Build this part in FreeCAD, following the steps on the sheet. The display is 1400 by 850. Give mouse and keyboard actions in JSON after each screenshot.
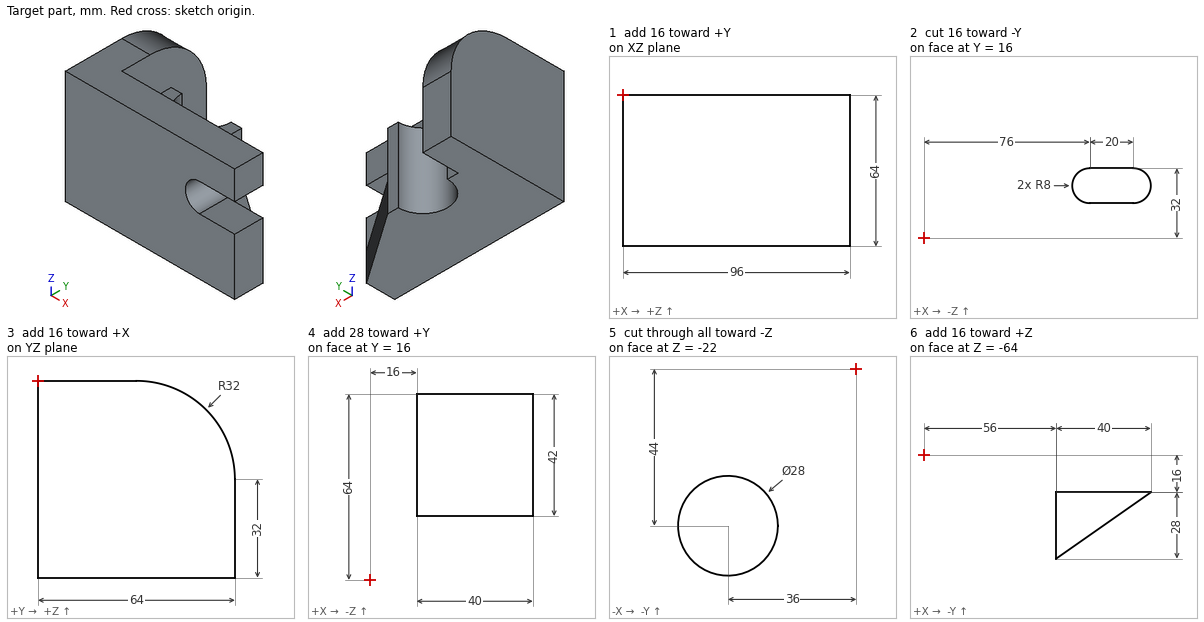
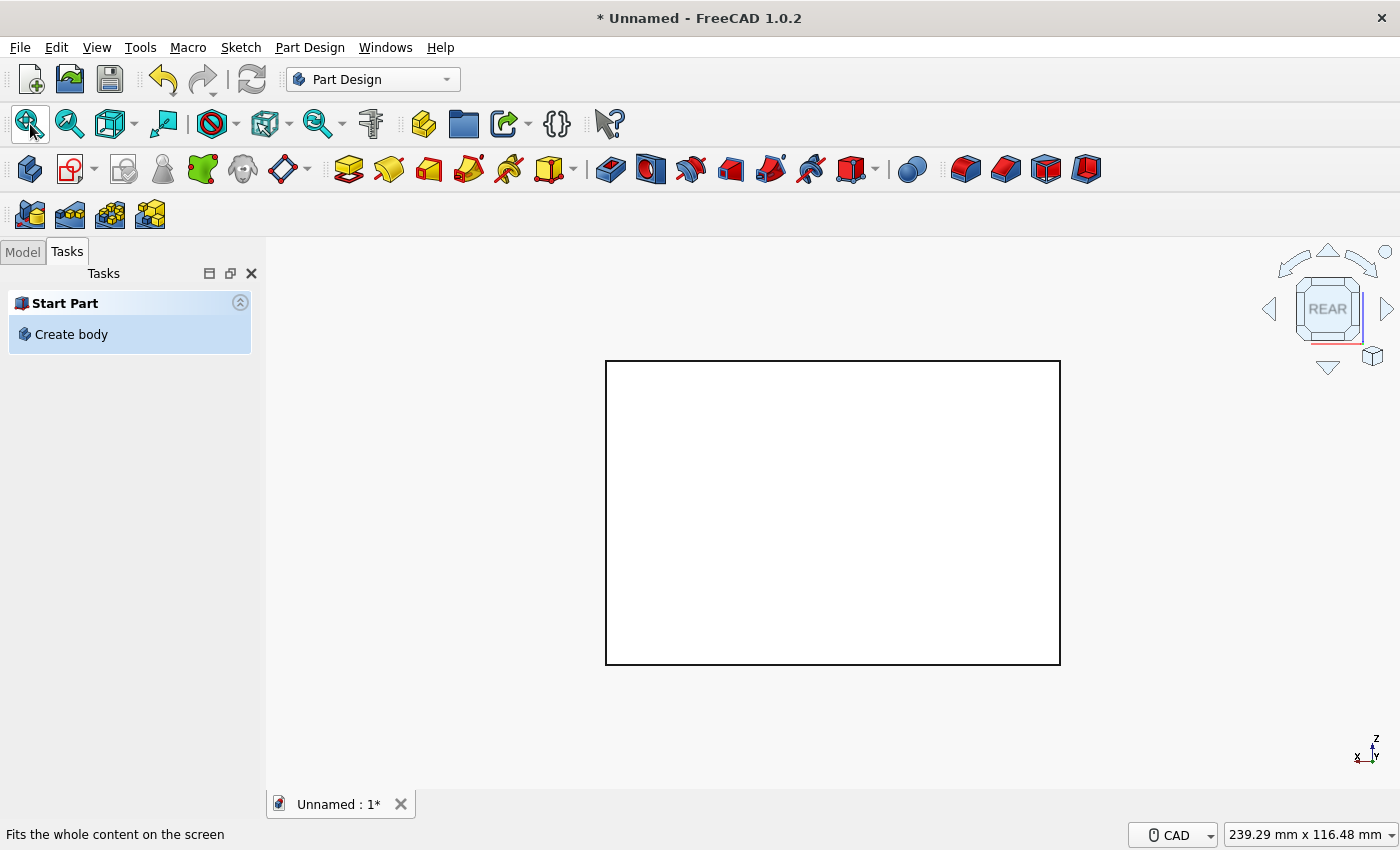
{"action": "left_click", "coordinate": [768, 512]}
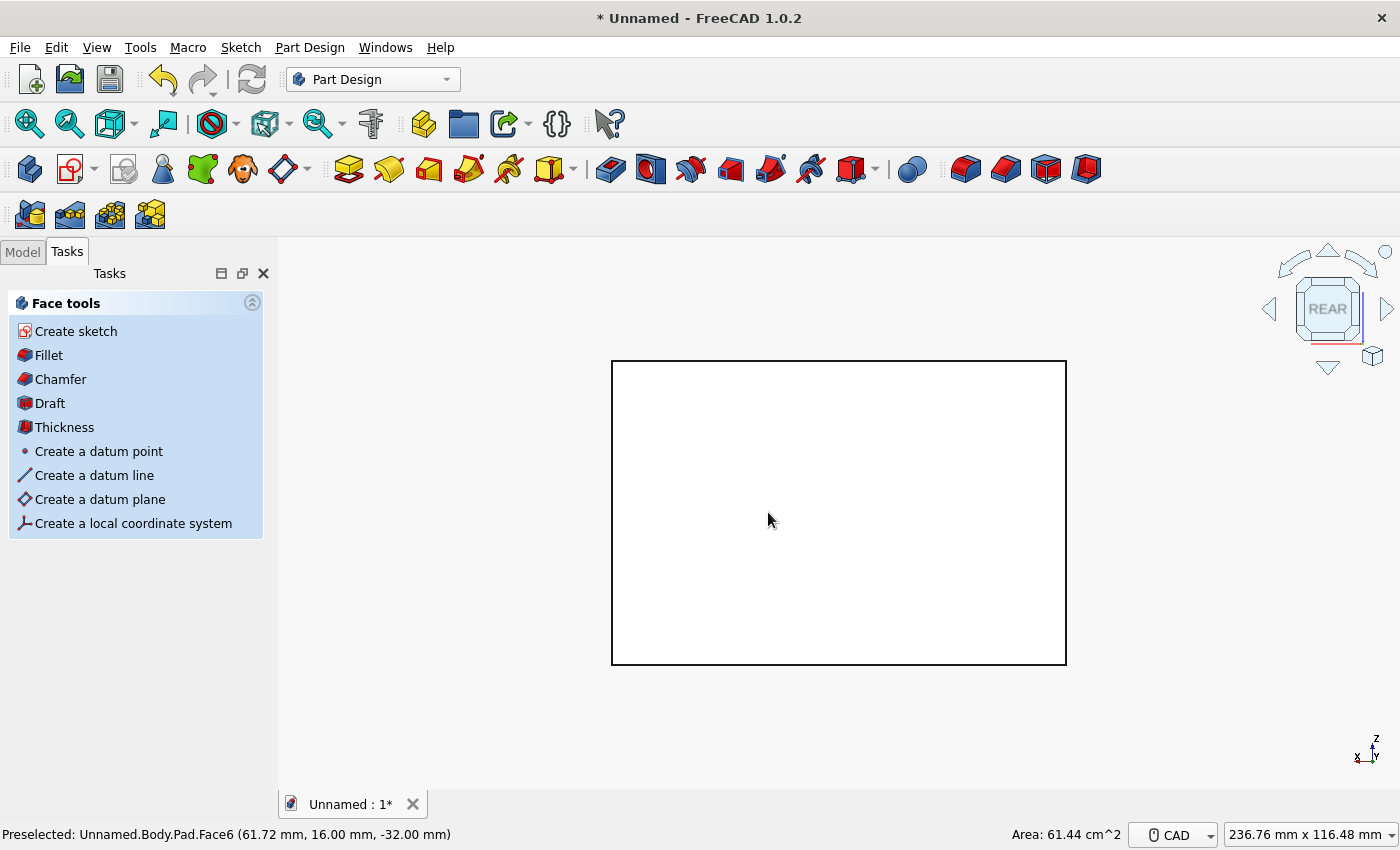
{"action": "left_click", "coordinate": [70, 170]}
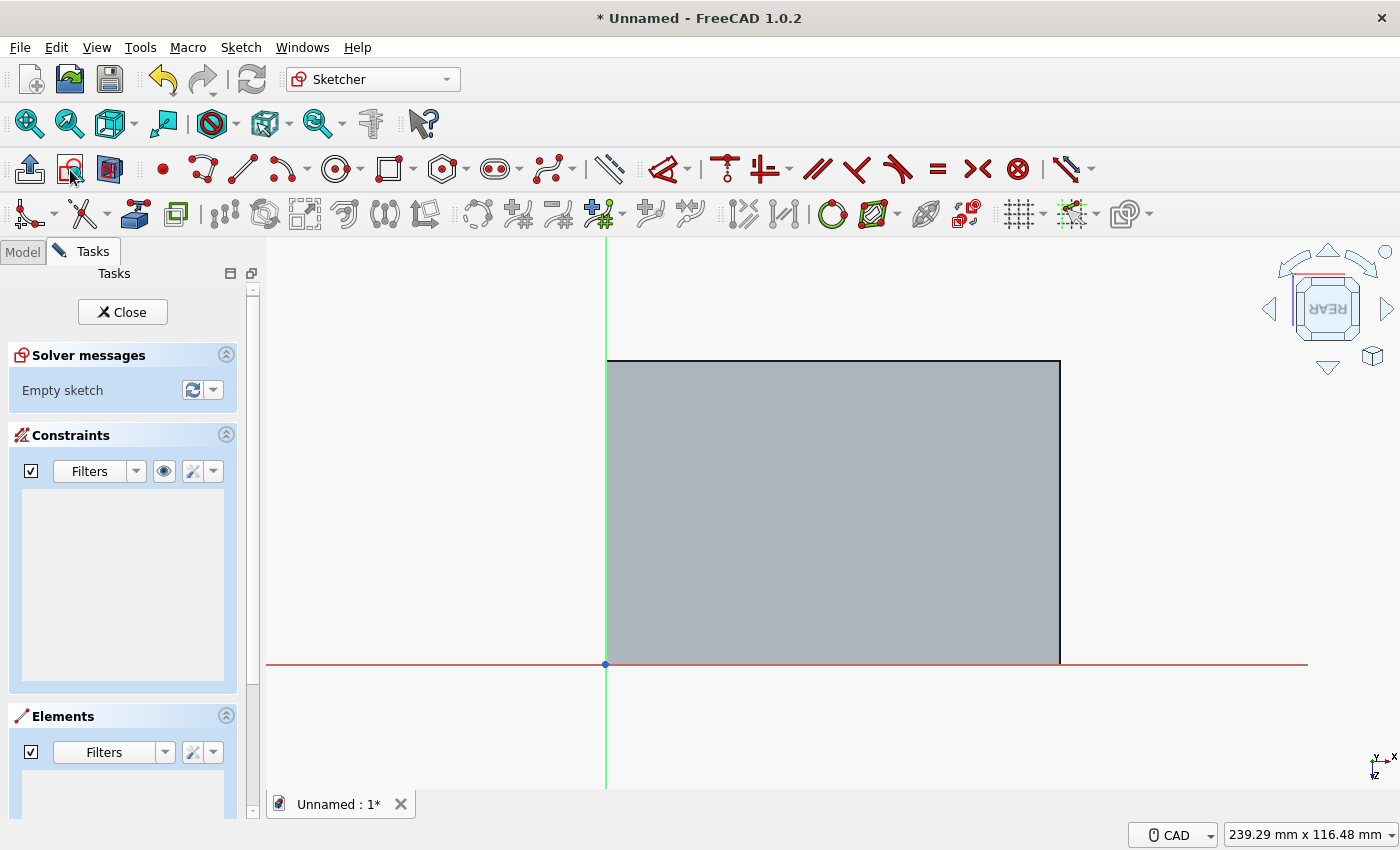
{"action": "scroll", "coordinate": [1094, 563], "scroll_direction": "up", "scroll_amount": 7}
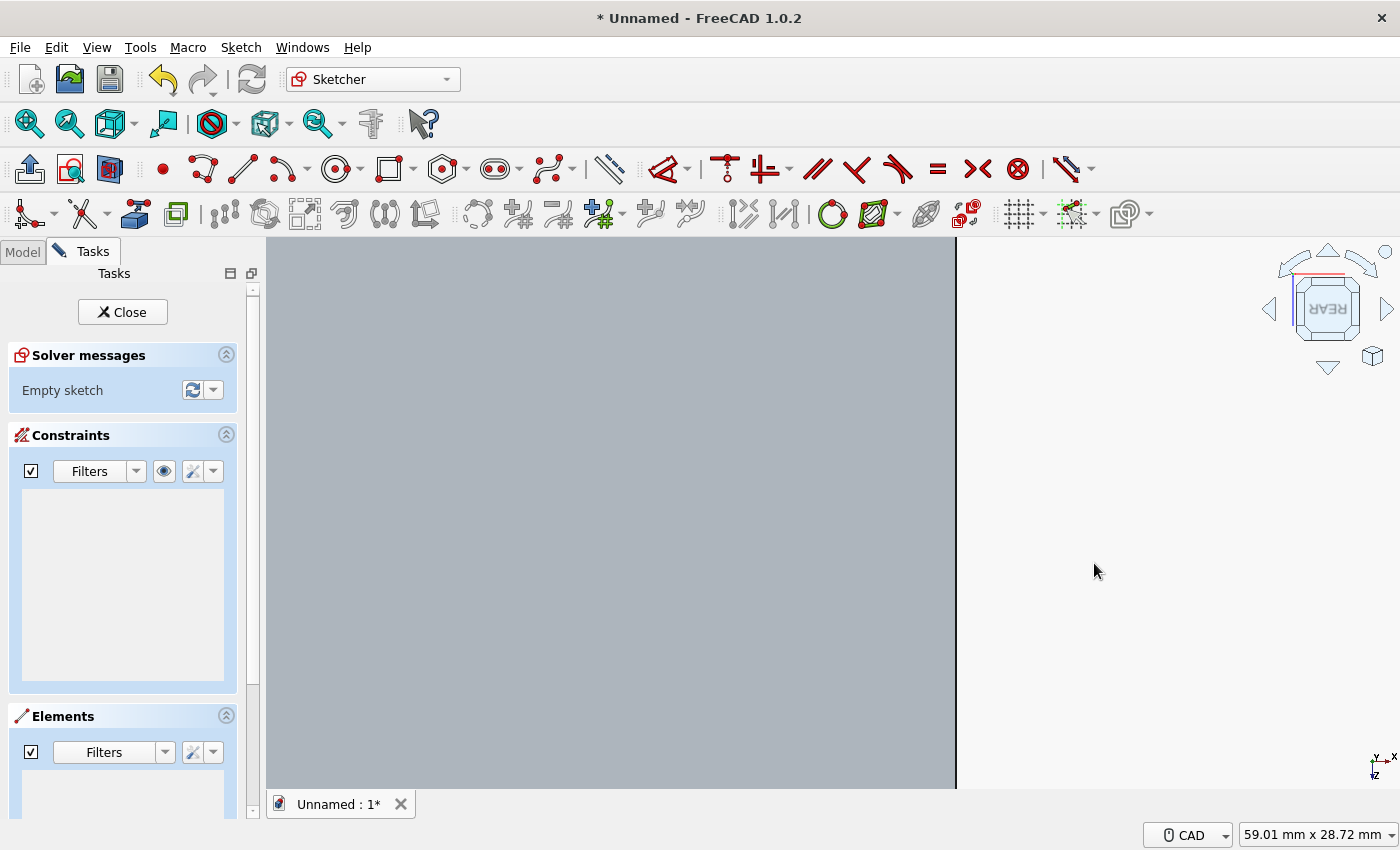
{"action": "left_click", "coordinate": [496, 170]}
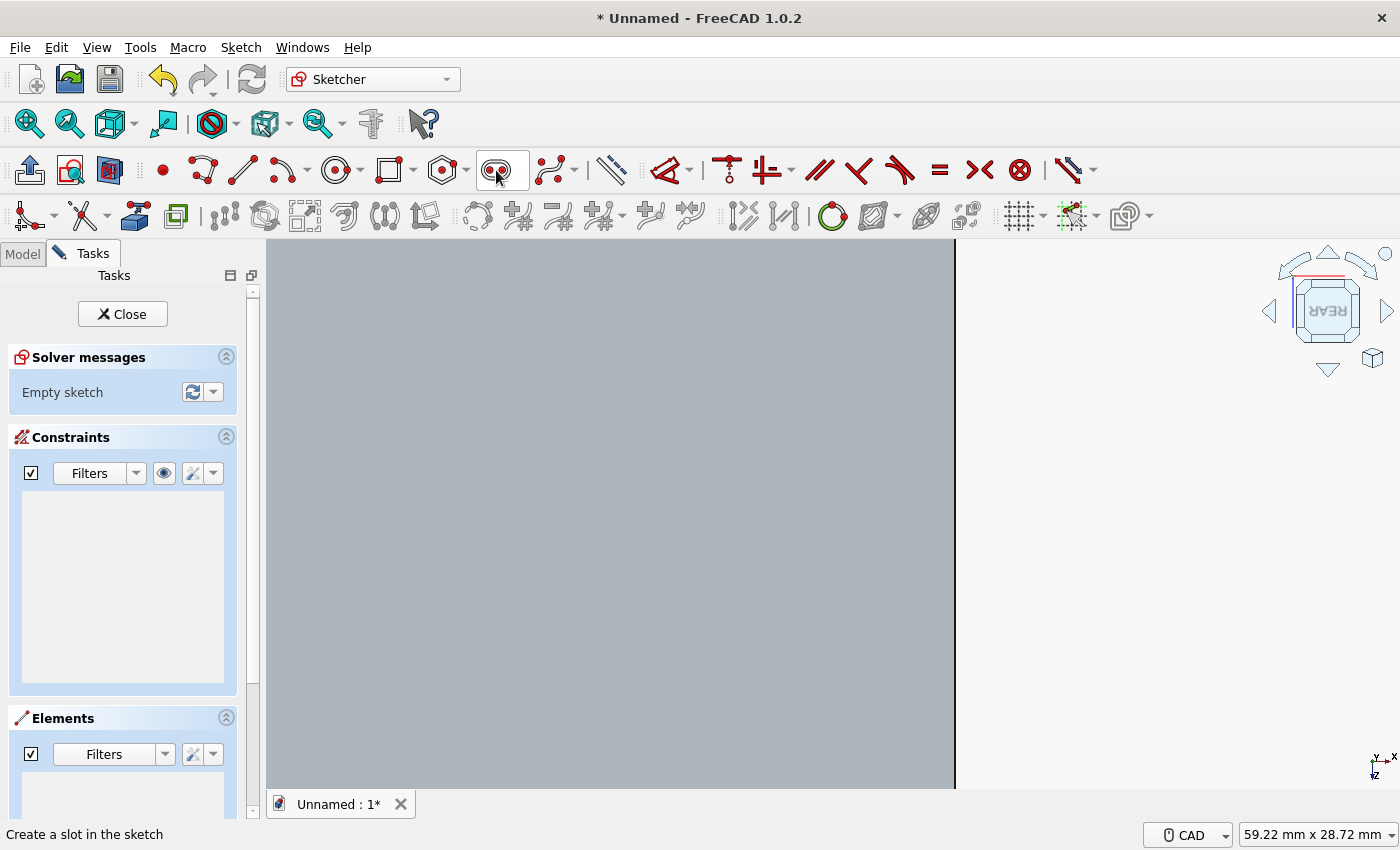
{"action": "left_click", "coordinate": [572, 513]}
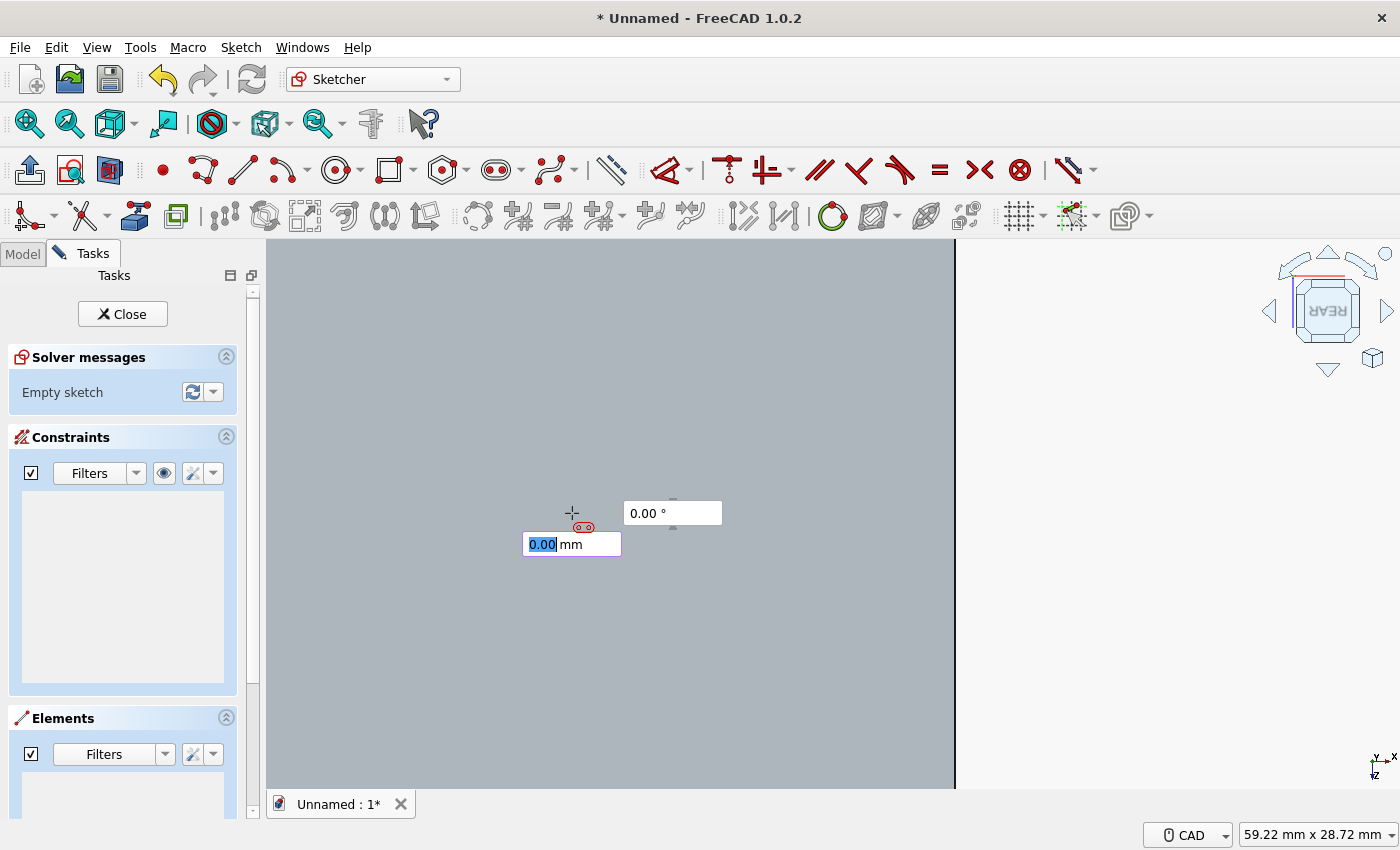
{"action": "left_click", "coordinate": [955, 513]}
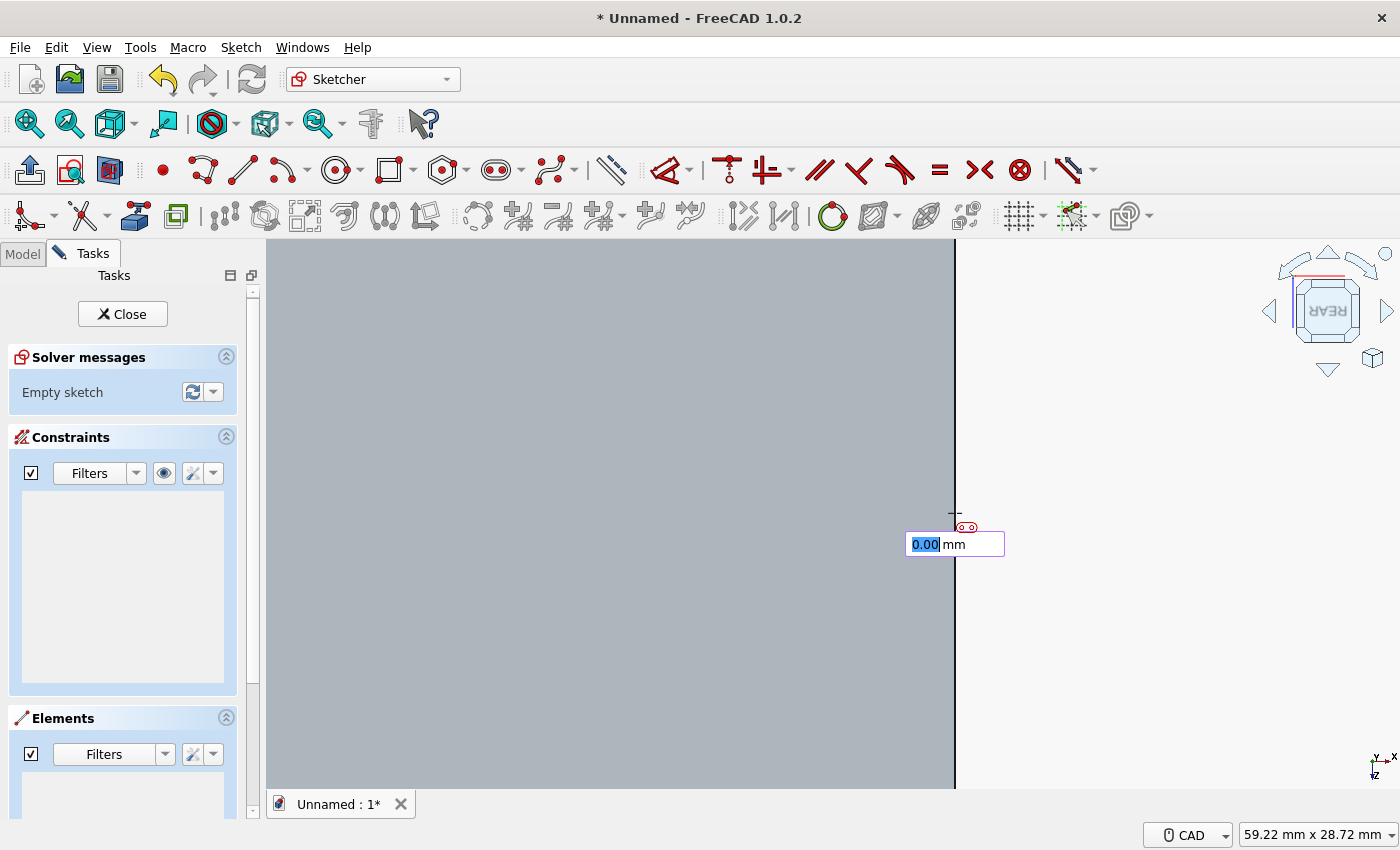
{"action": "left_click", "coordinate": [764, 666]}
{"action": "key", "text": "Escape"}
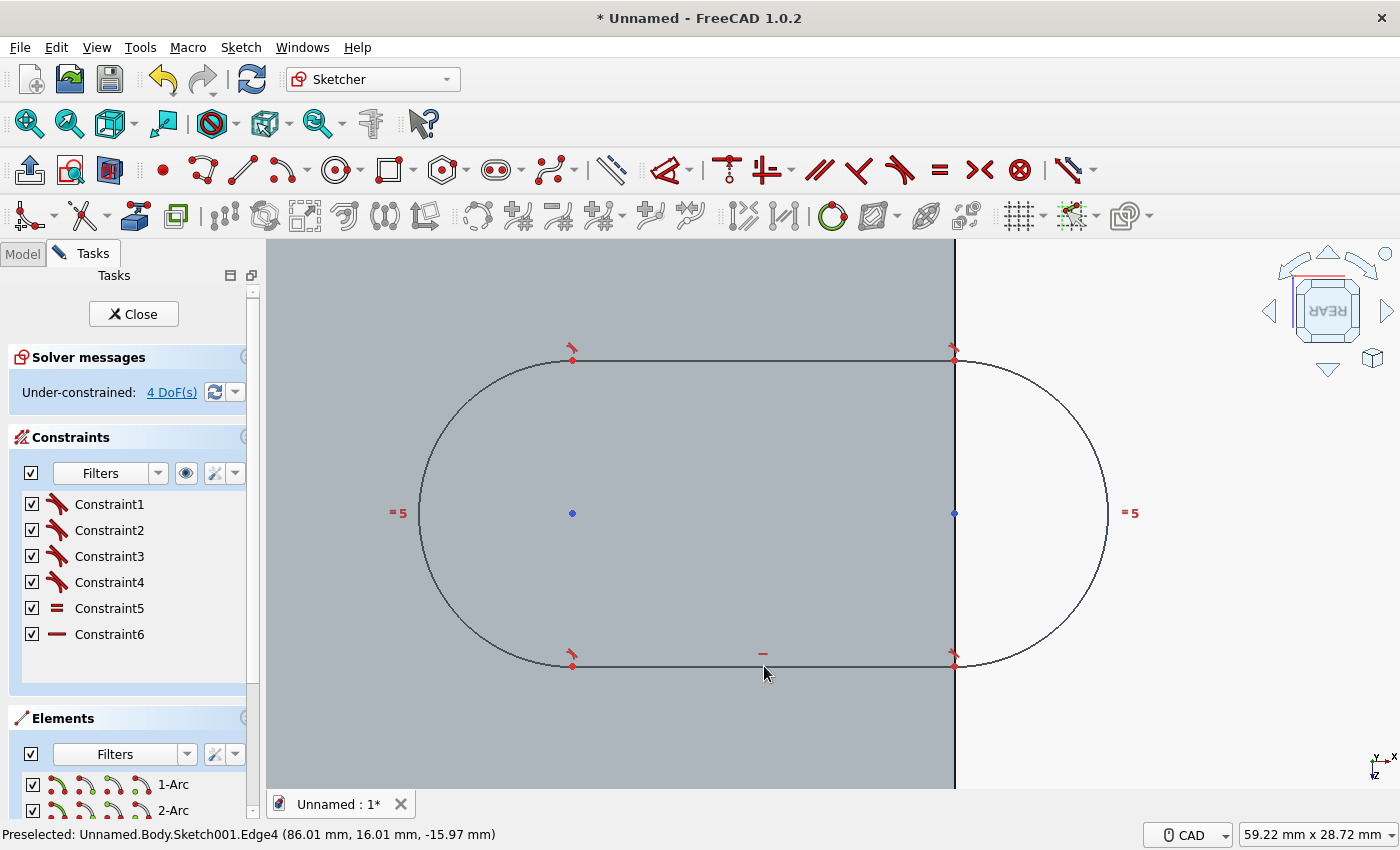
{"action": "left_click", "coordinate": [666, 170]}